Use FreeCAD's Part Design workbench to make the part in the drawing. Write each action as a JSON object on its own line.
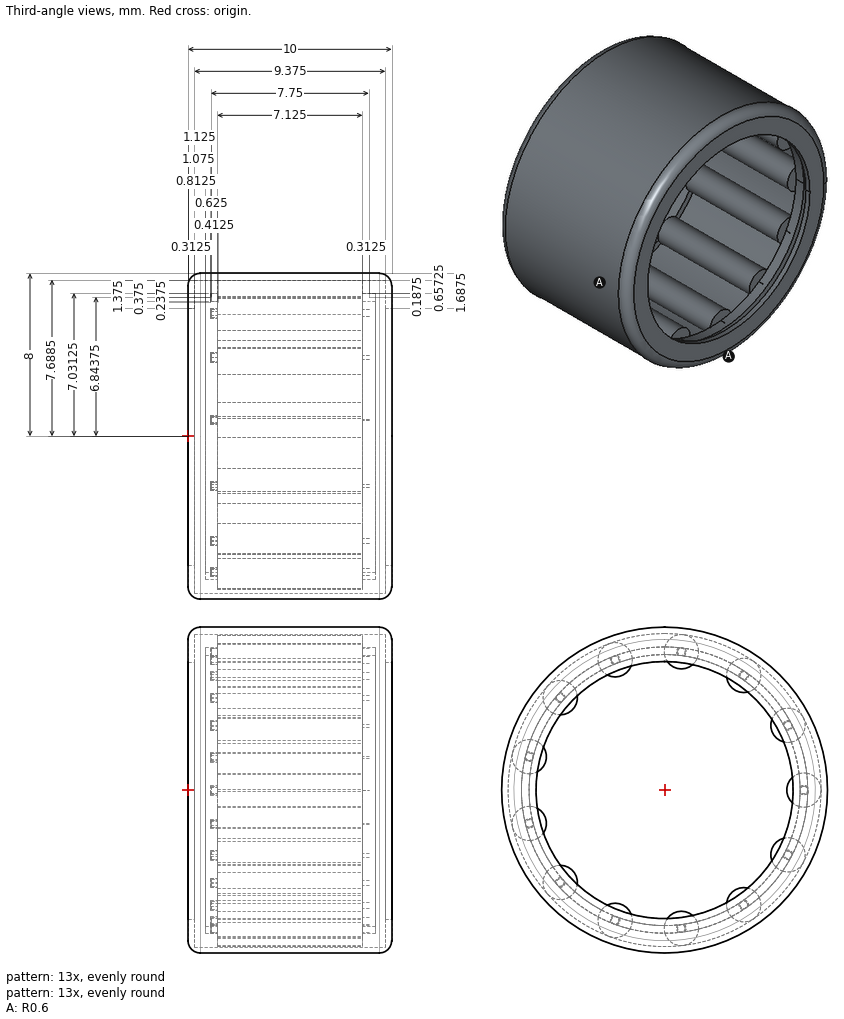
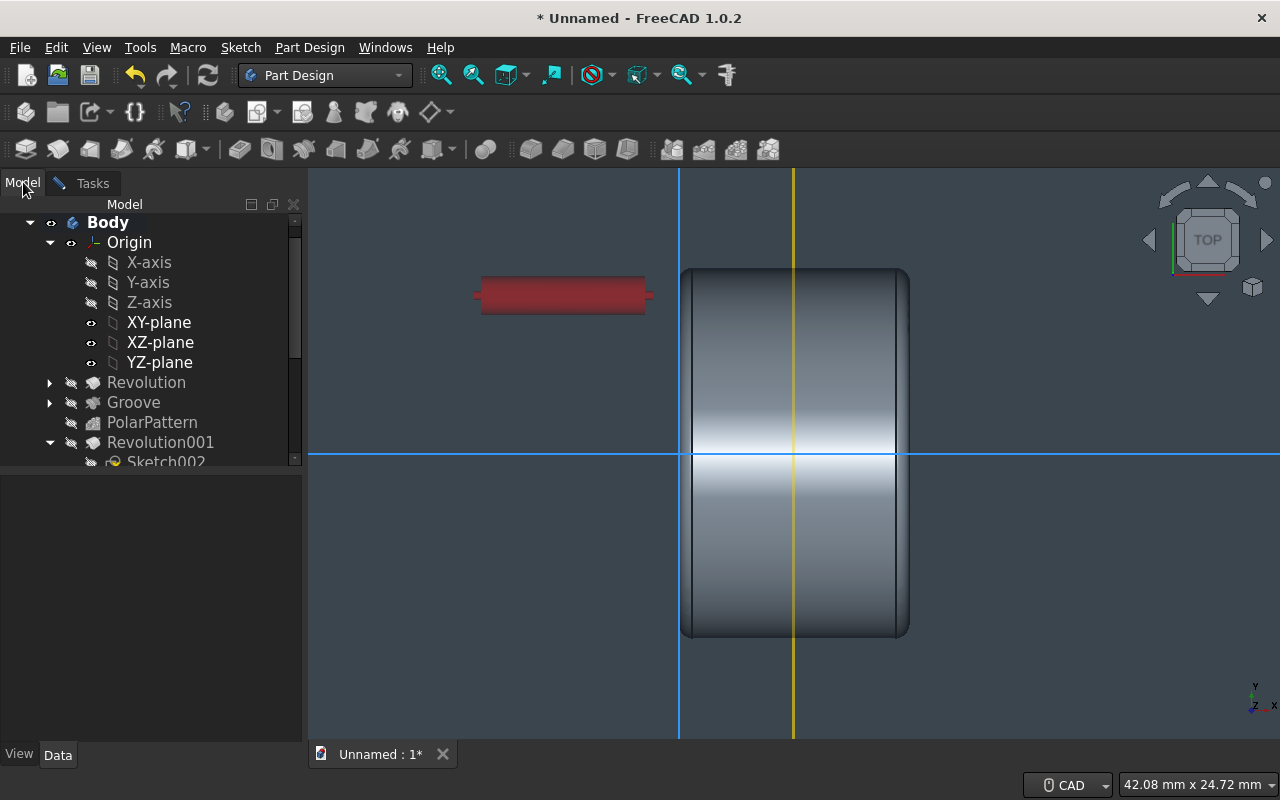
{"action": "scroll", "coordinate": [120, 338], "scroll_direction": "down", "scroll_amount": 3}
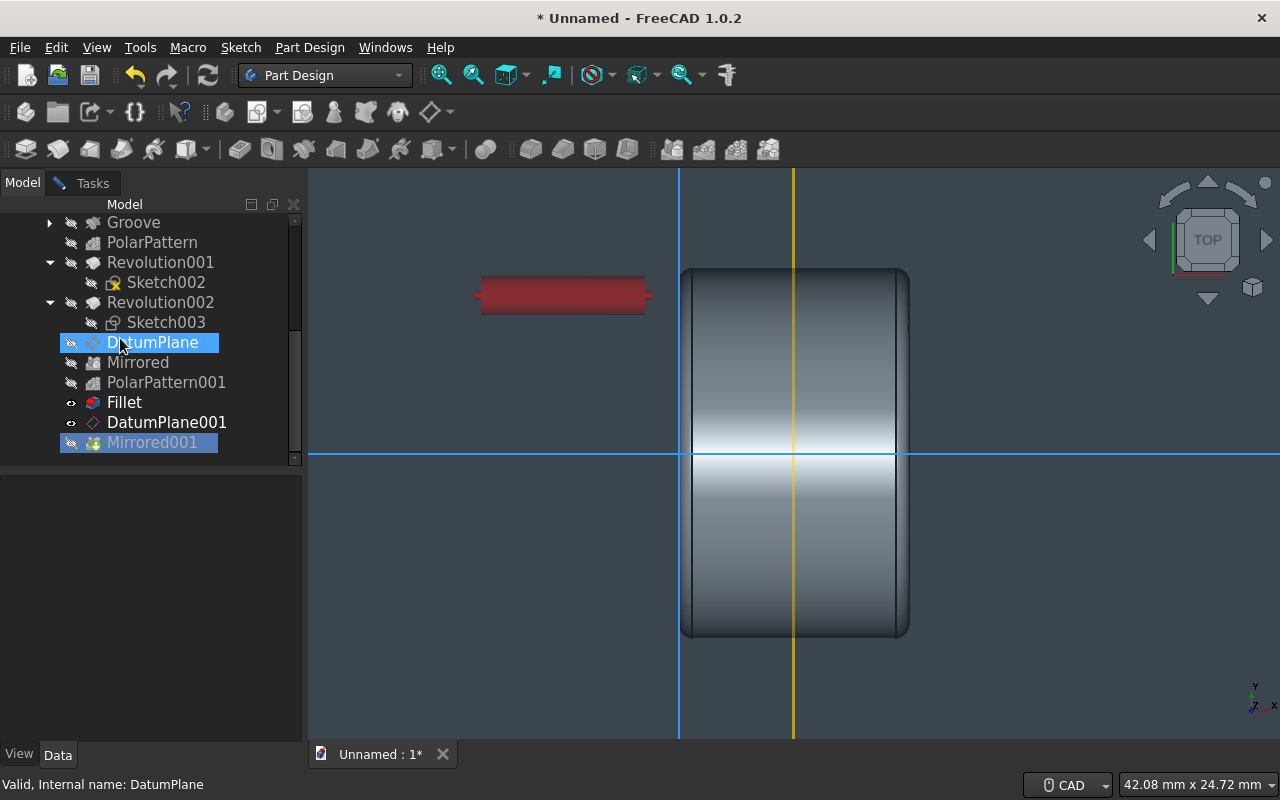
{"action": "left_click", "coordinate": [116, 423]}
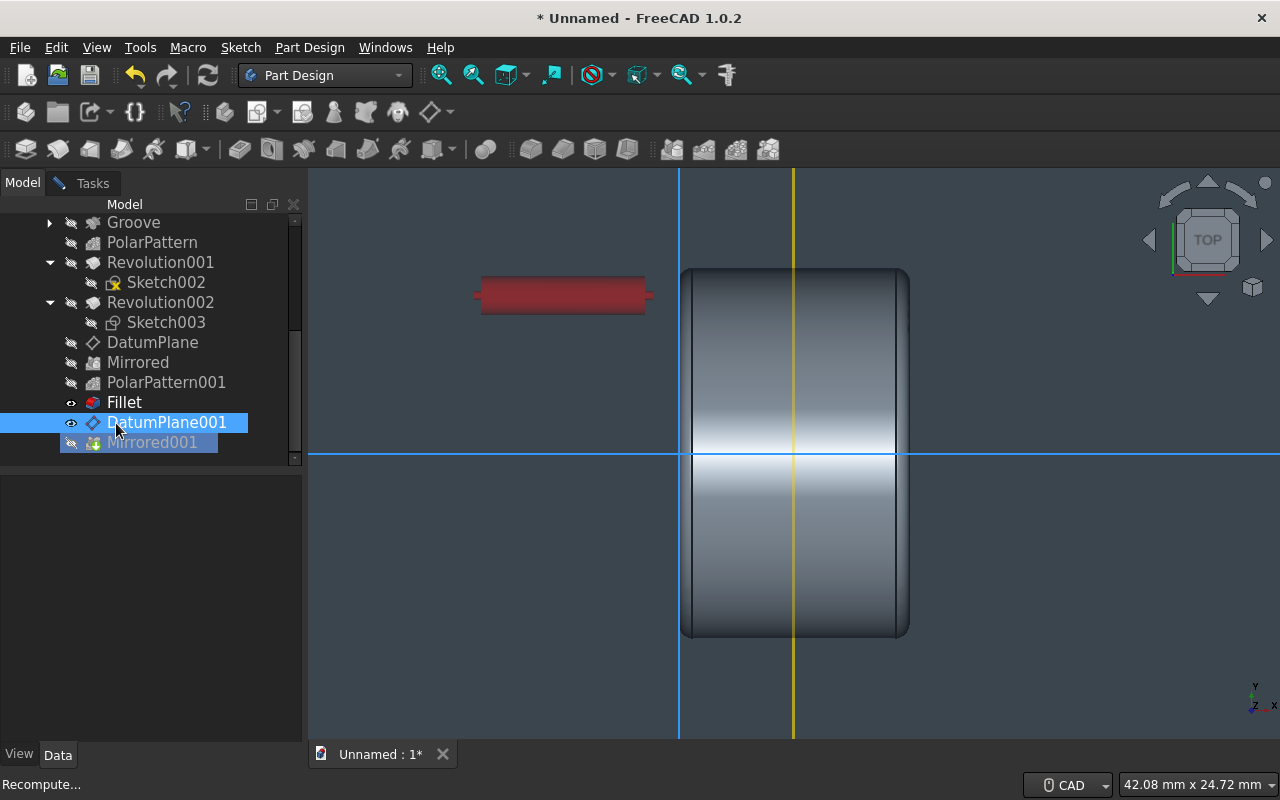
{"action": "left_click", "coordinate": [84, 182]}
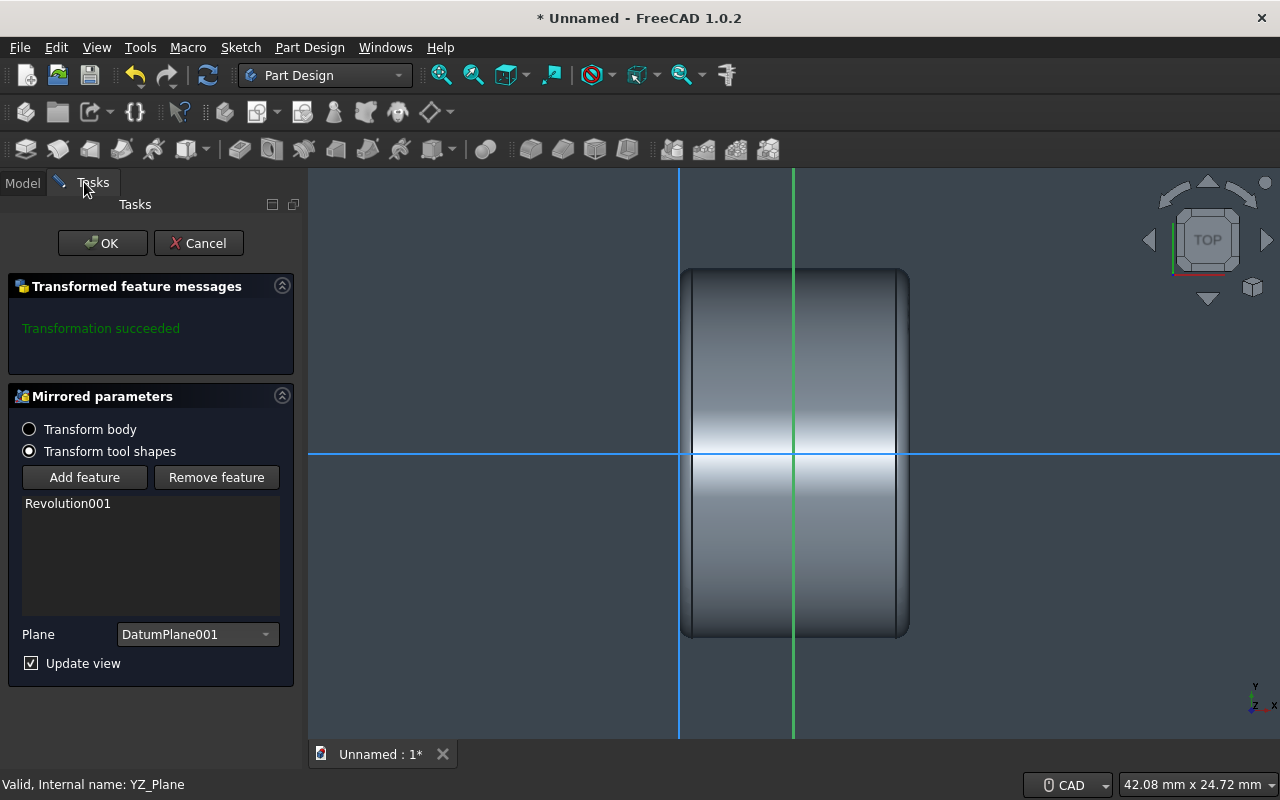
{"action": "left_click", "coordinate": [103, 243]}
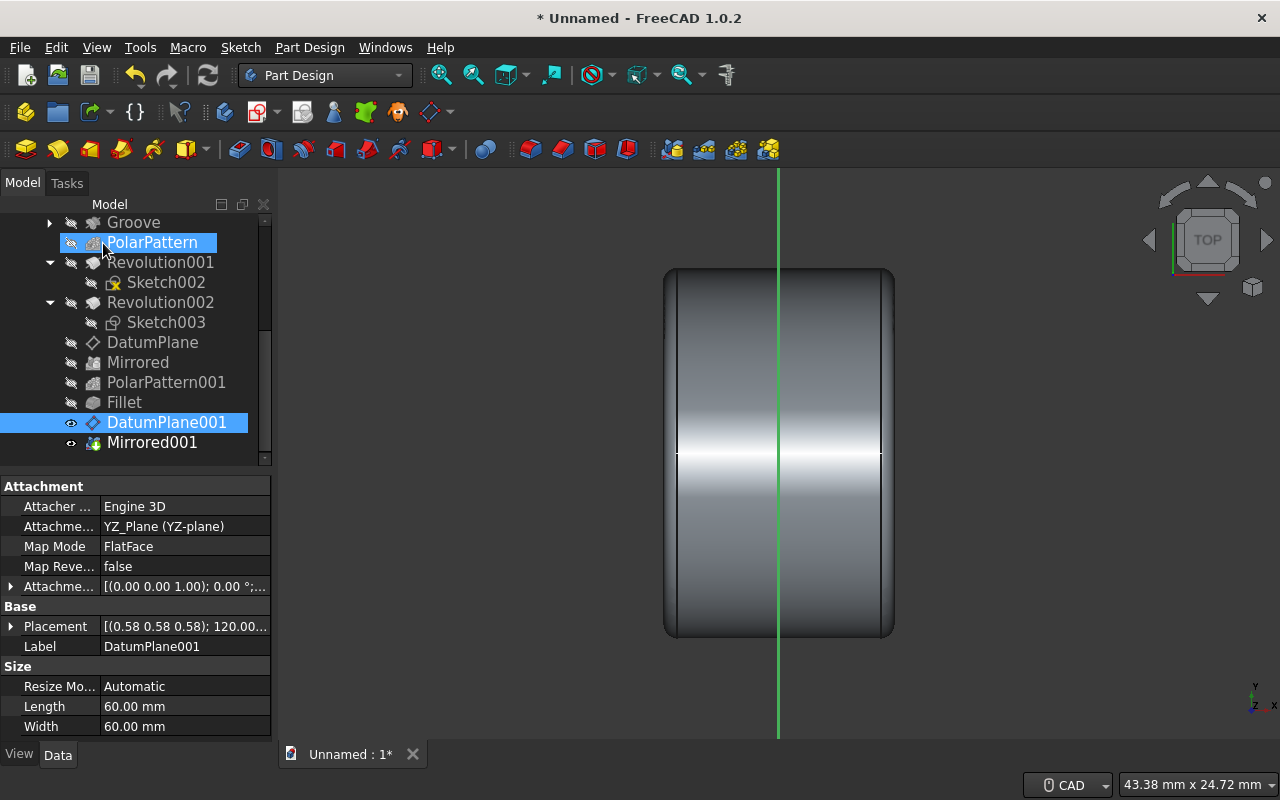
{"action": "left_click", "coordinate": [116, 423]}
{"action": "key", "text": "space"}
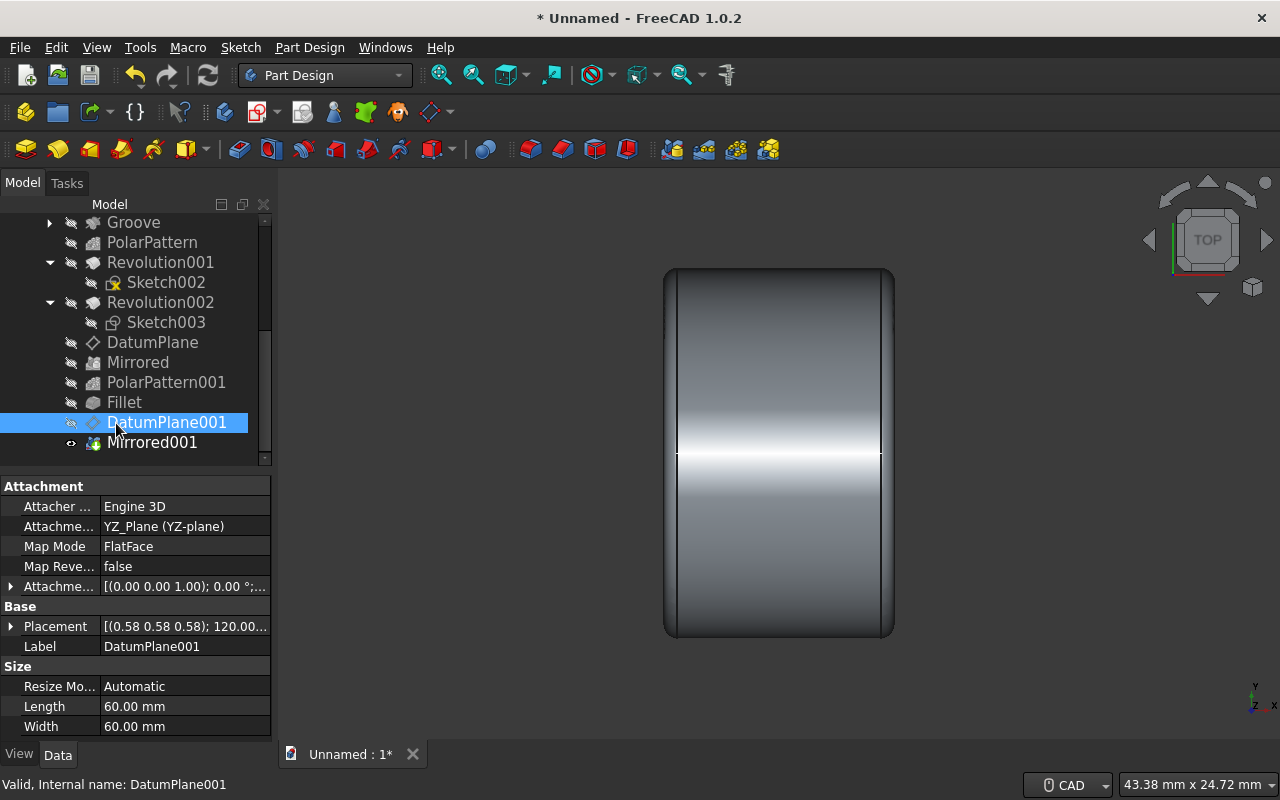
{"action": "key", "text": "0"}